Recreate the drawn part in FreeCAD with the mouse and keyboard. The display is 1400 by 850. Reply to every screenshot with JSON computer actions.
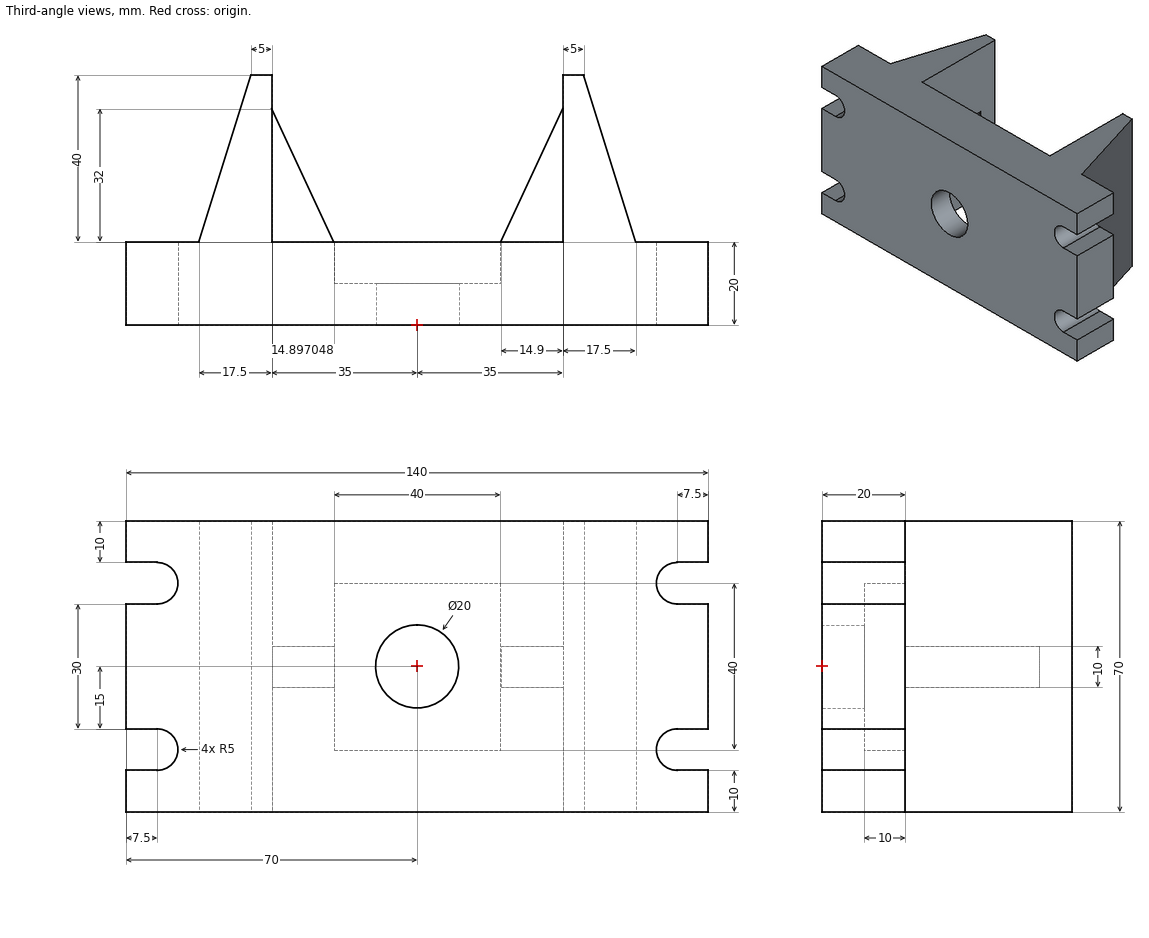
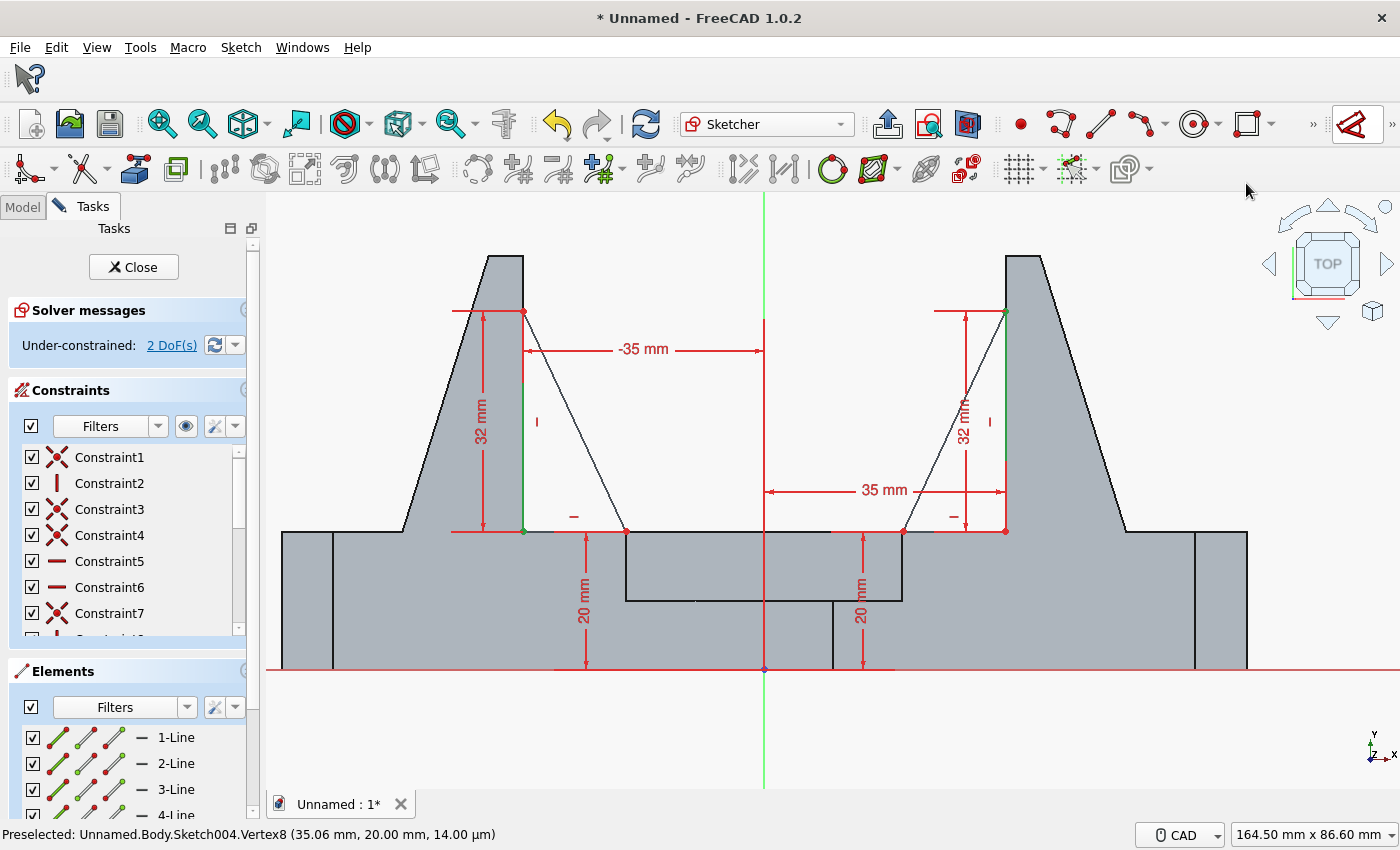
{"action": "left_click", "coordinate": [934, 532]}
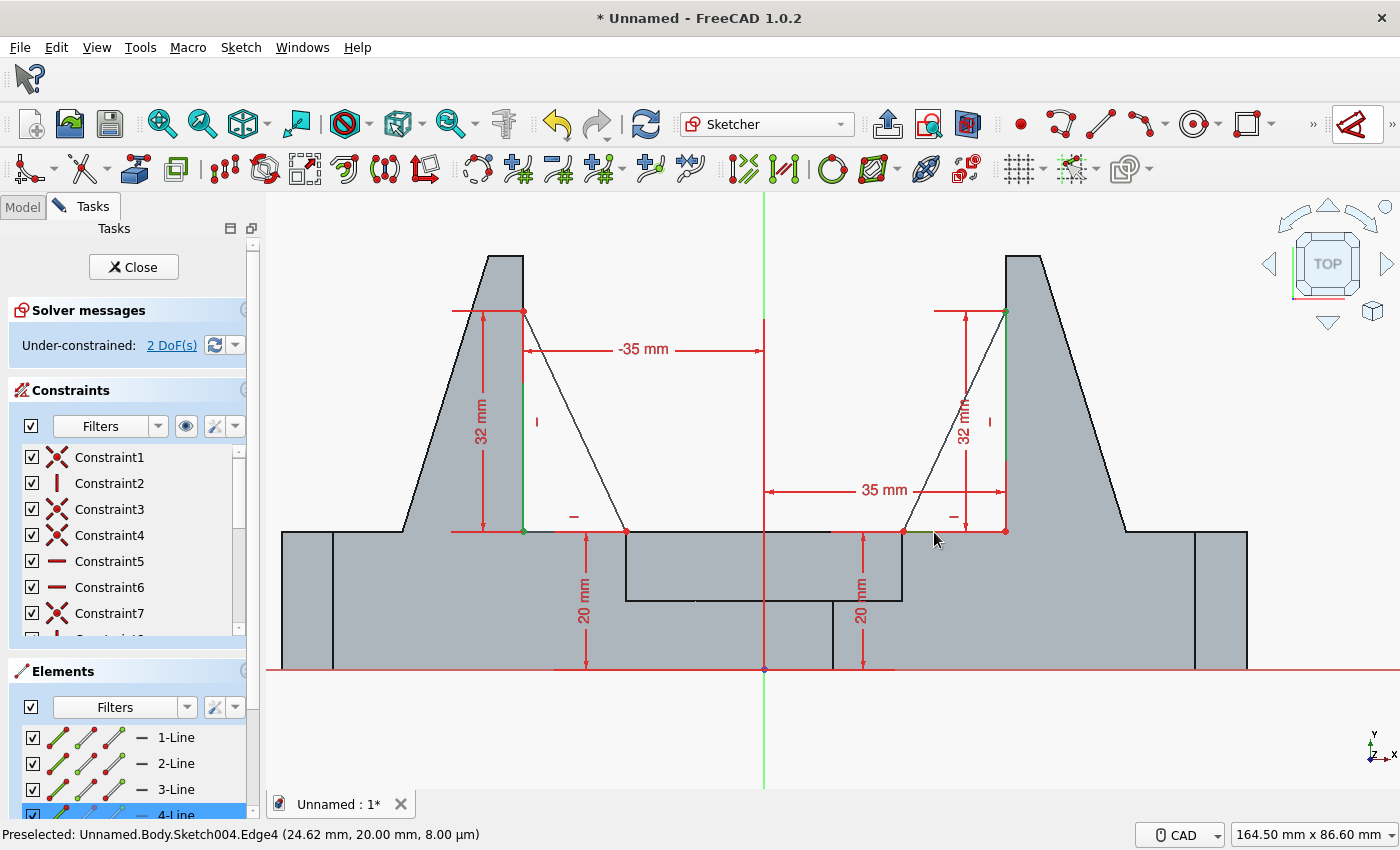
{"action": "key", "text": "l"}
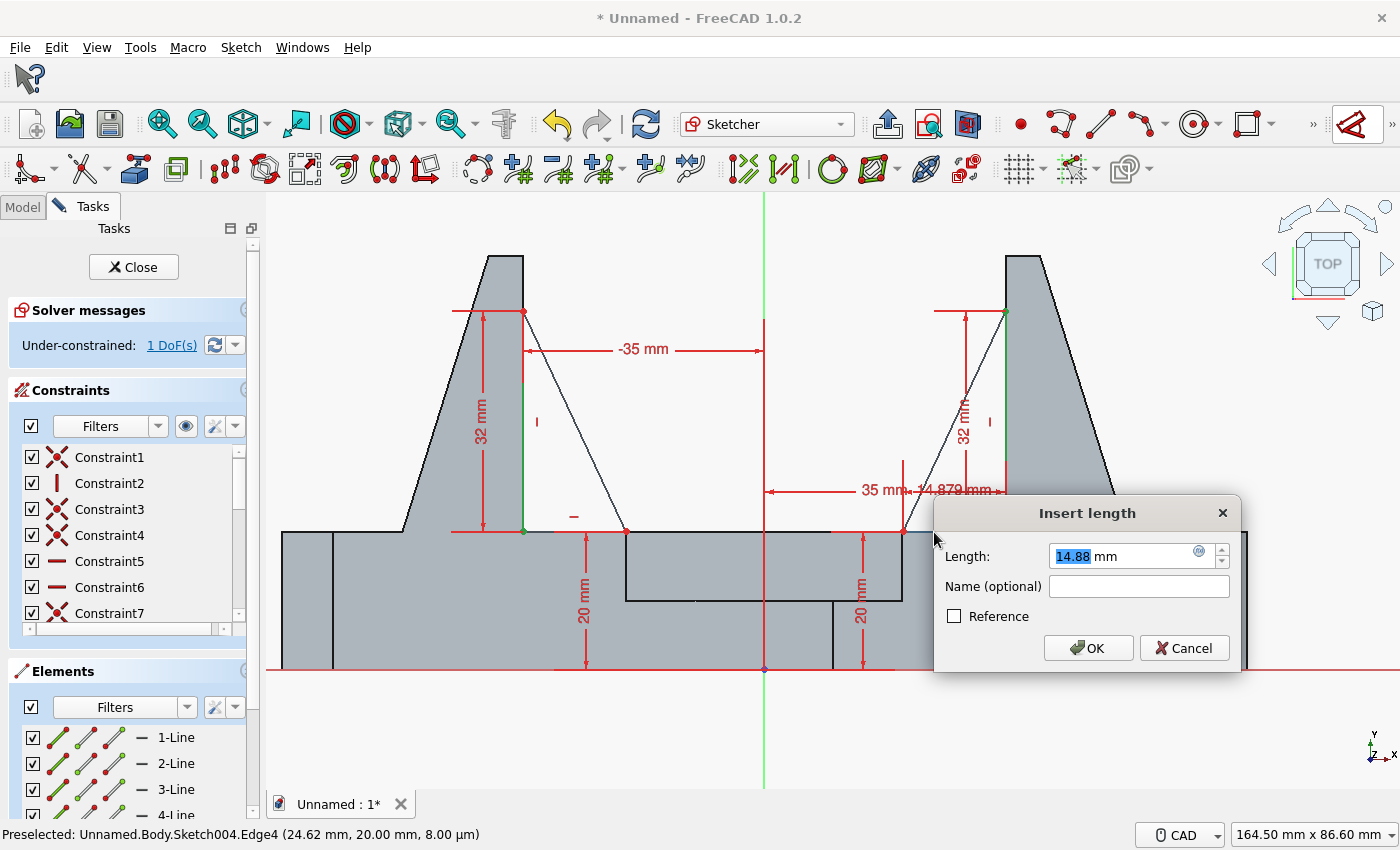
{"action": "type", "text": "14.9"}
{"action": "key", "text": "Return"}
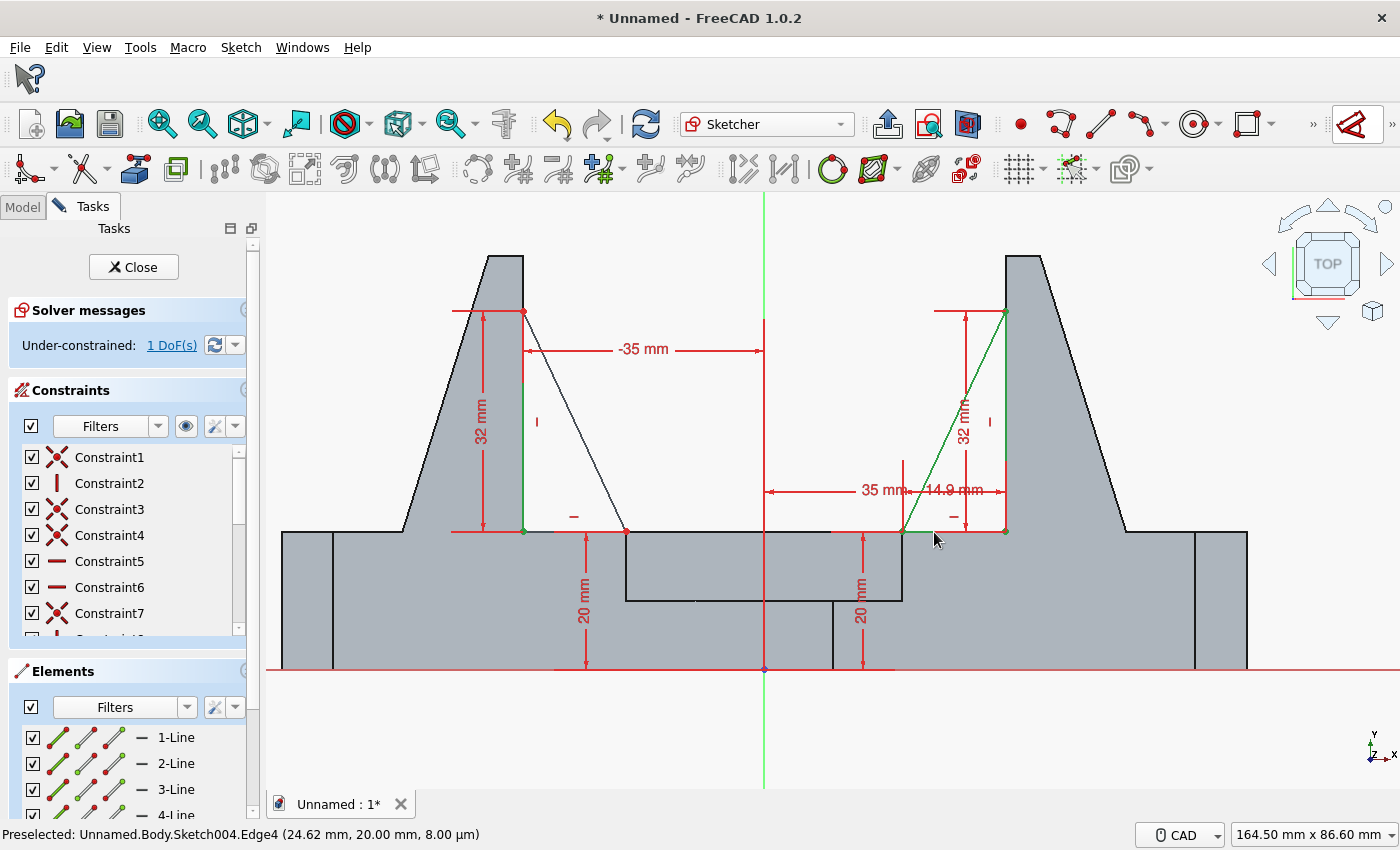
{"action": "left_click", "coordinate": [554, 532]}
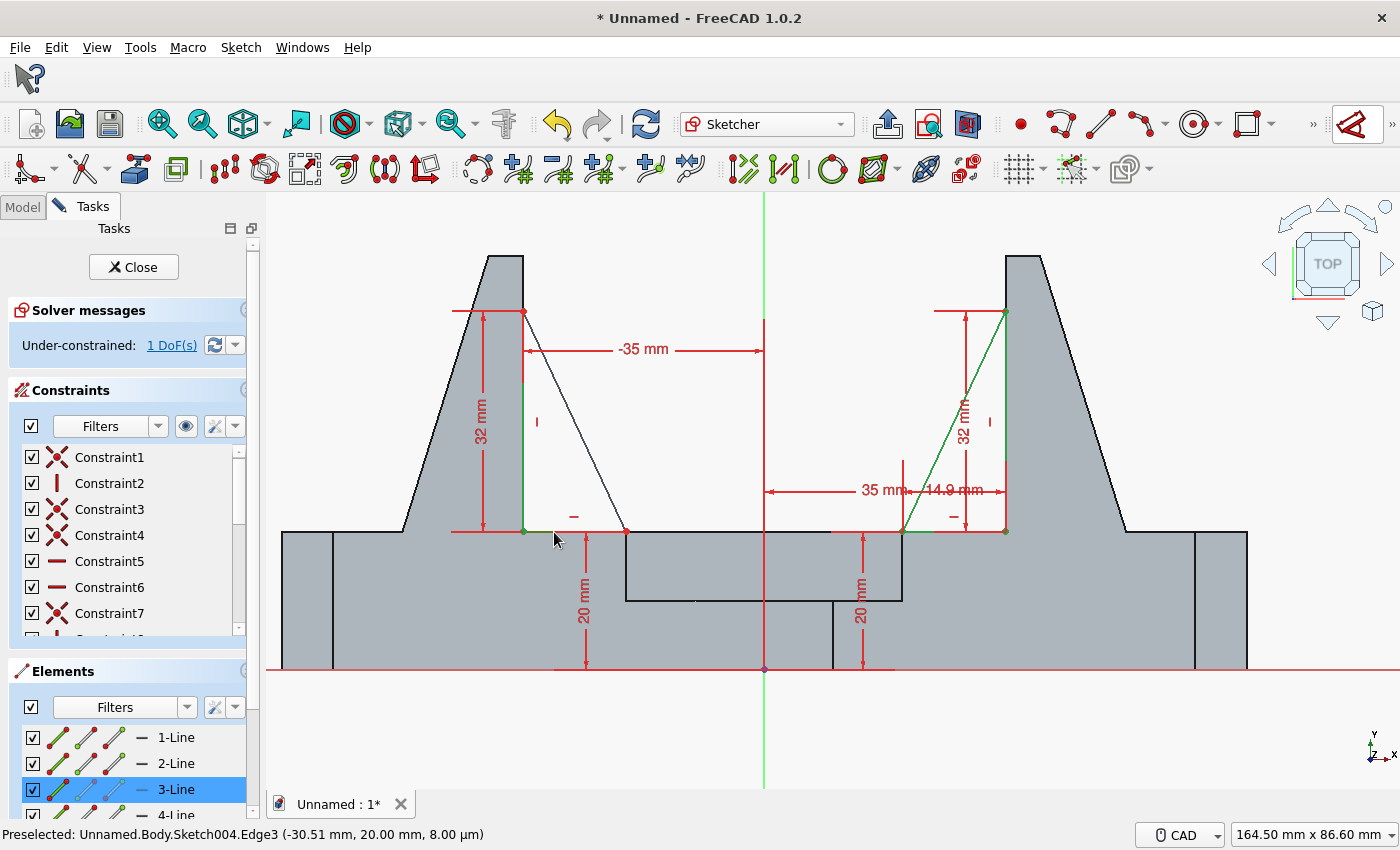
{"action": "left_click", "coordinate": [1378, 124]}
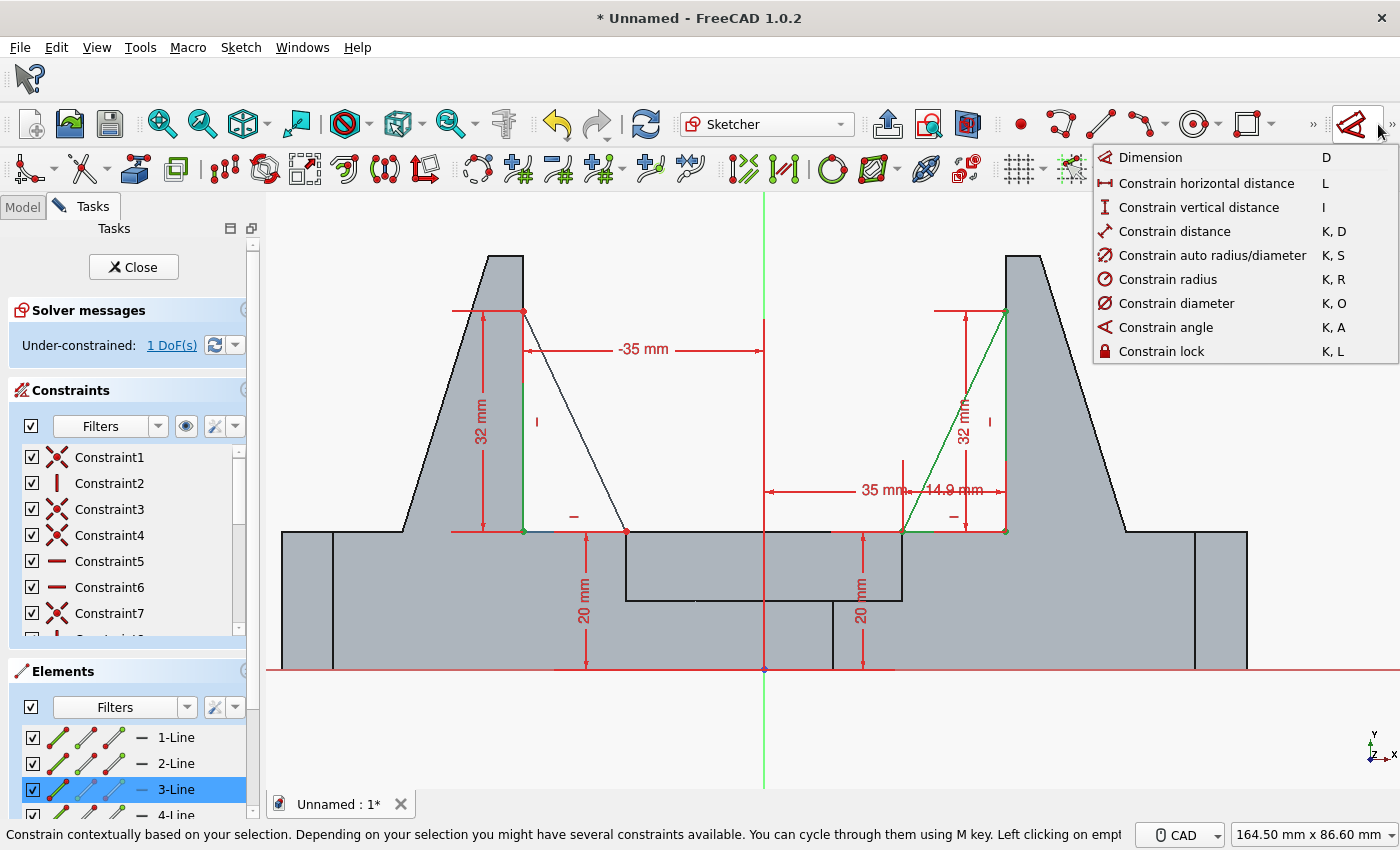
{"action": "left_click", "coordinate": [1246, 183]}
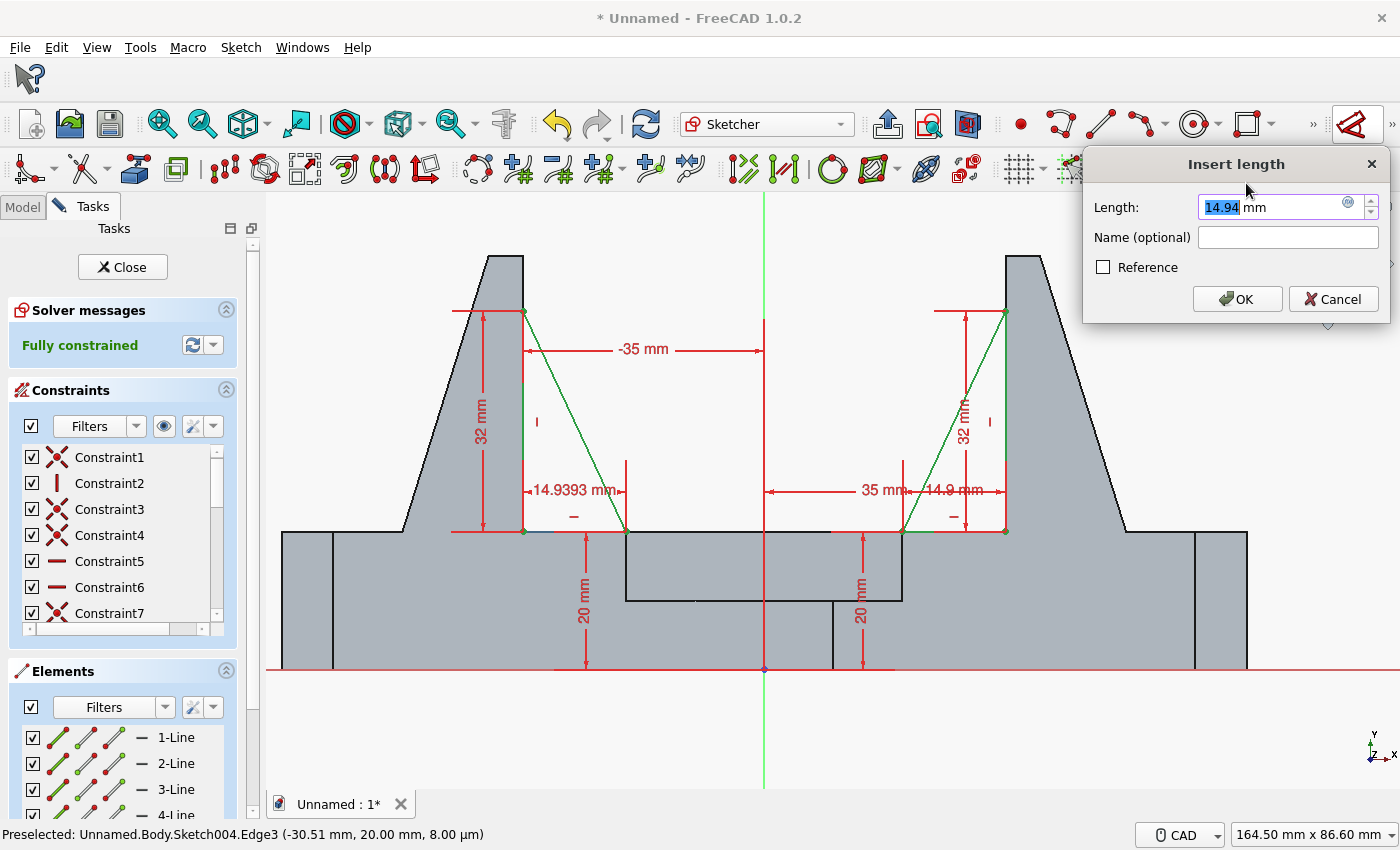
{"action": "type", "text": "14.897048"}
{"action": "key", "text": "Return"}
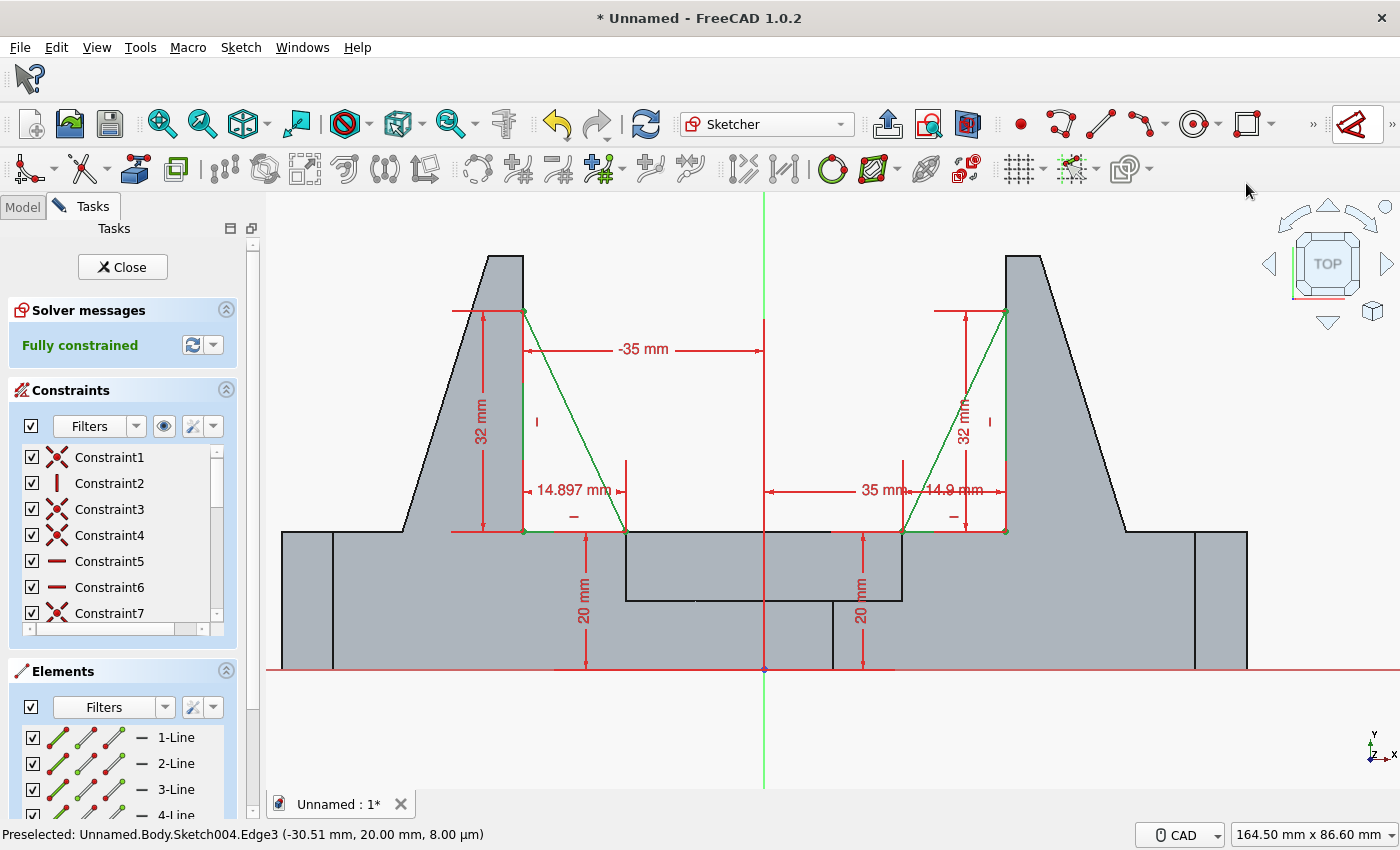
{"action": "left_click", "coordinate": [123, 267]}